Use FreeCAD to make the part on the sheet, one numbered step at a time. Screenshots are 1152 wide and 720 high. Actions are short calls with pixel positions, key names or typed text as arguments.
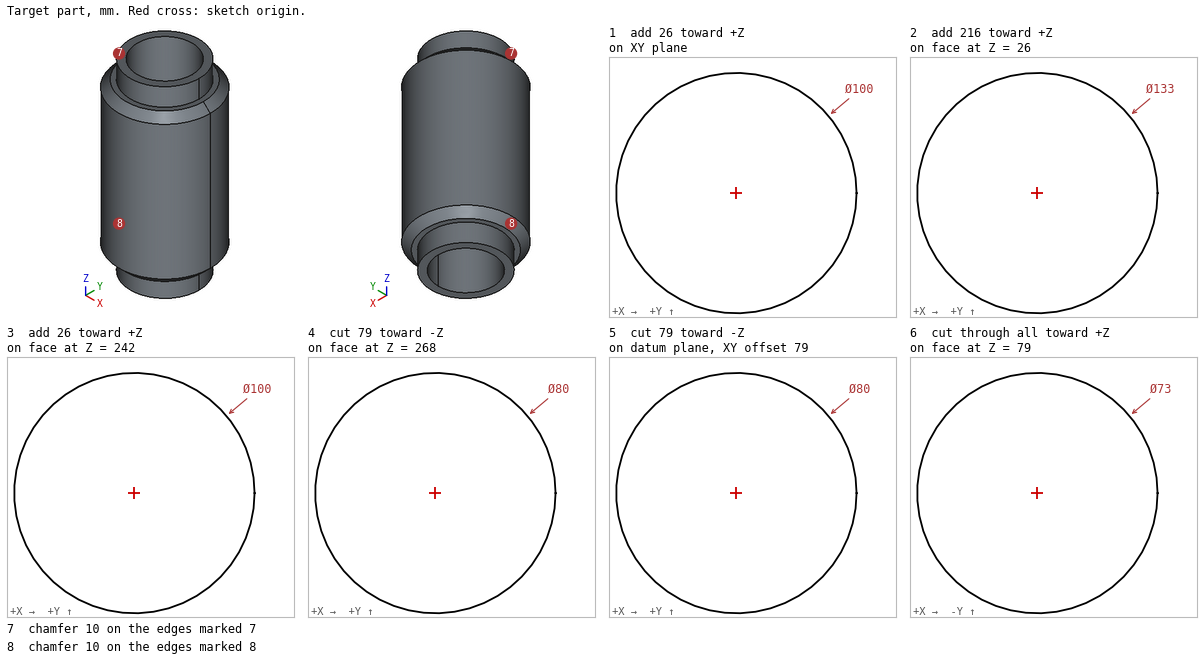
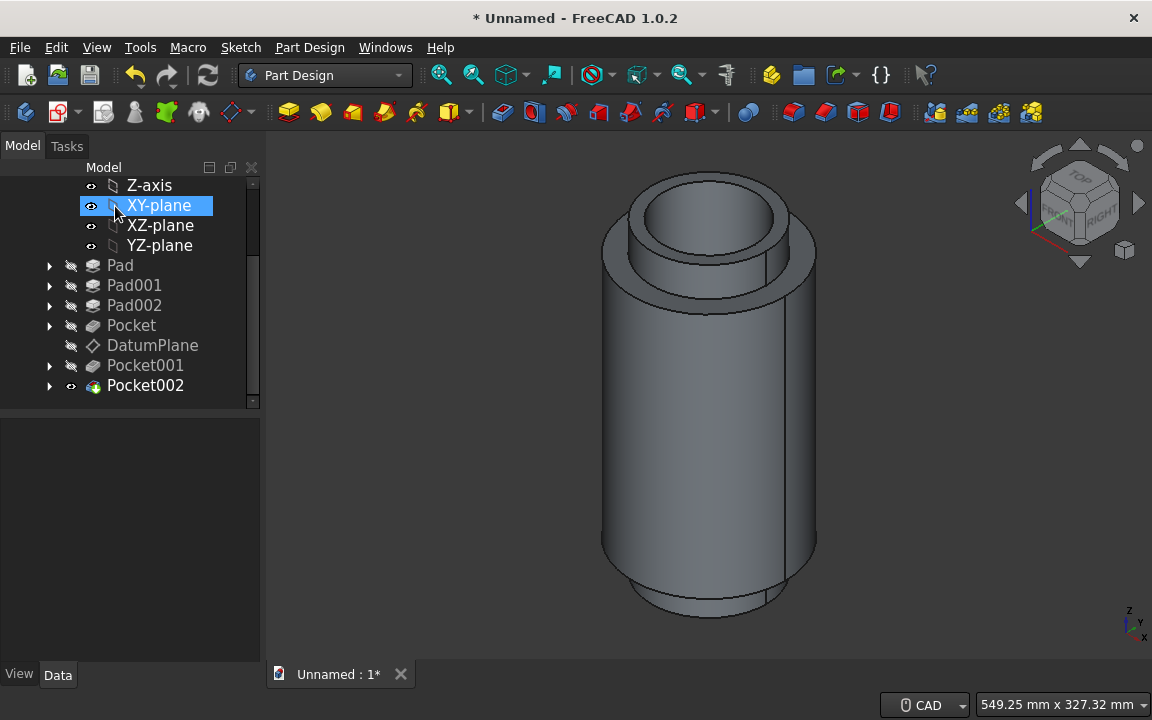
click(613, 280)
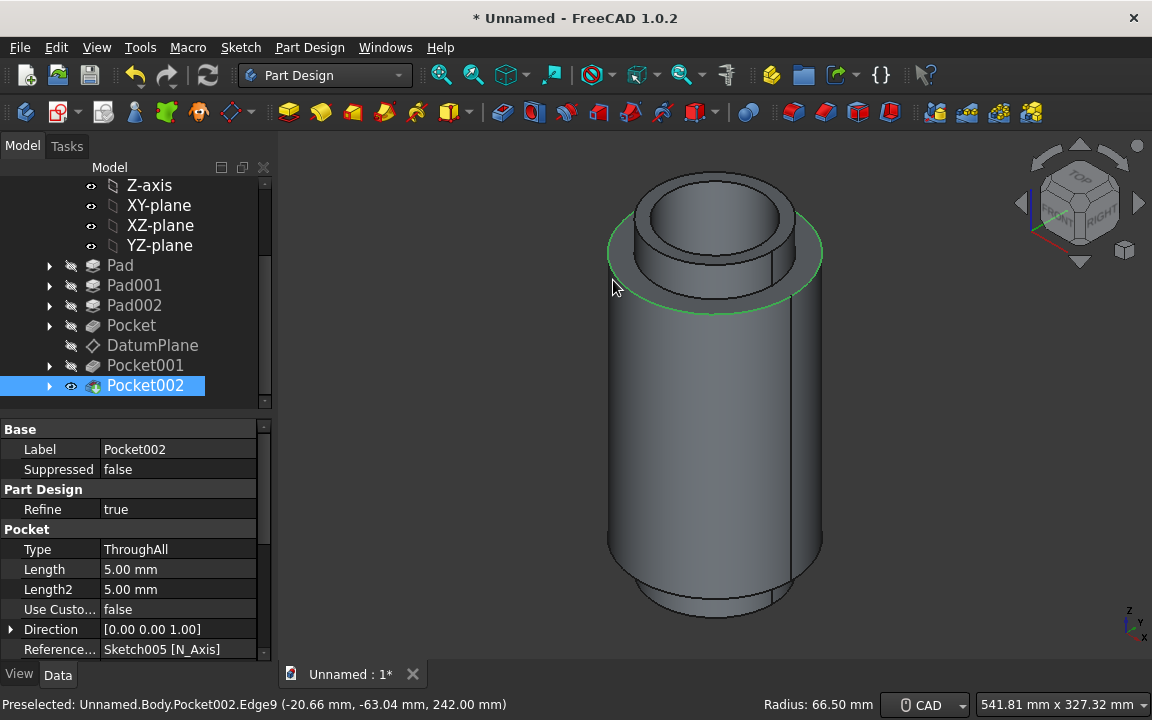
click(826, 112)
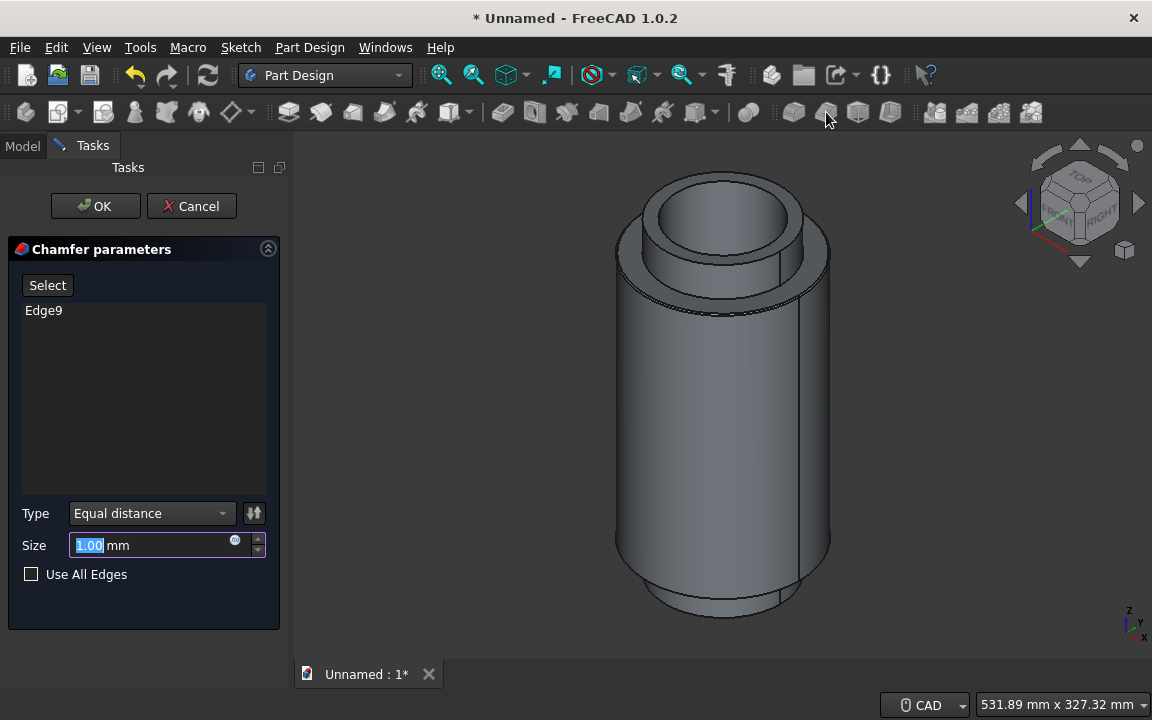
text(10)
key(Tab)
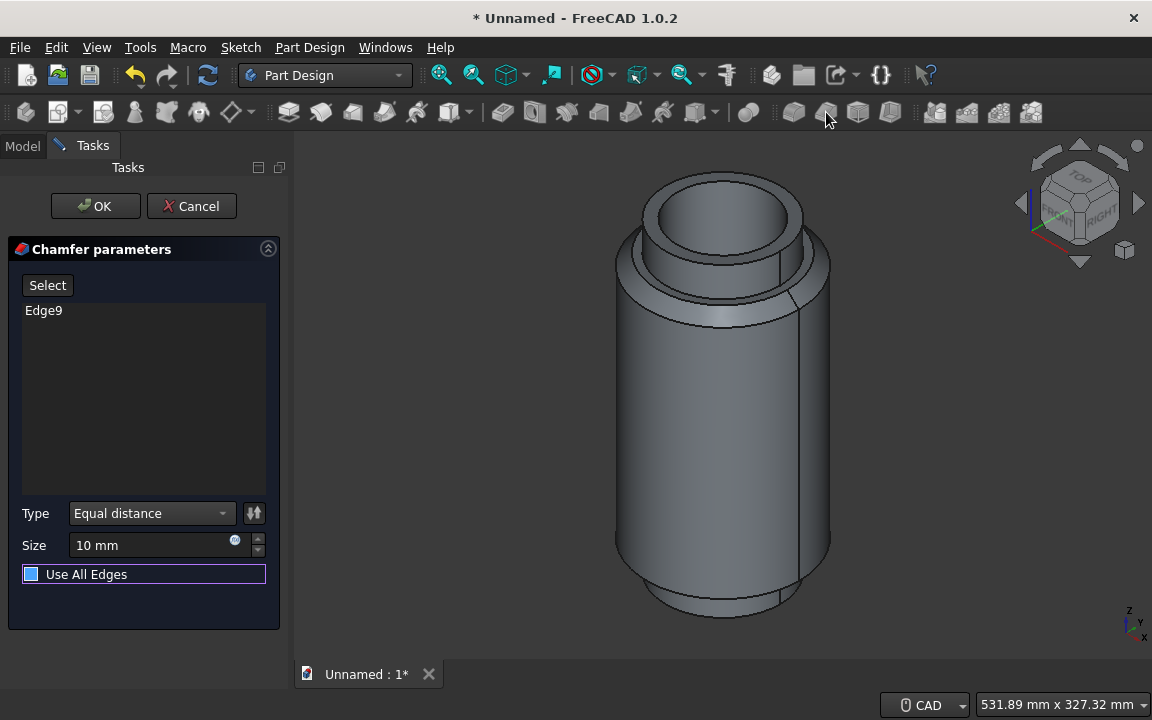
click(96, 206)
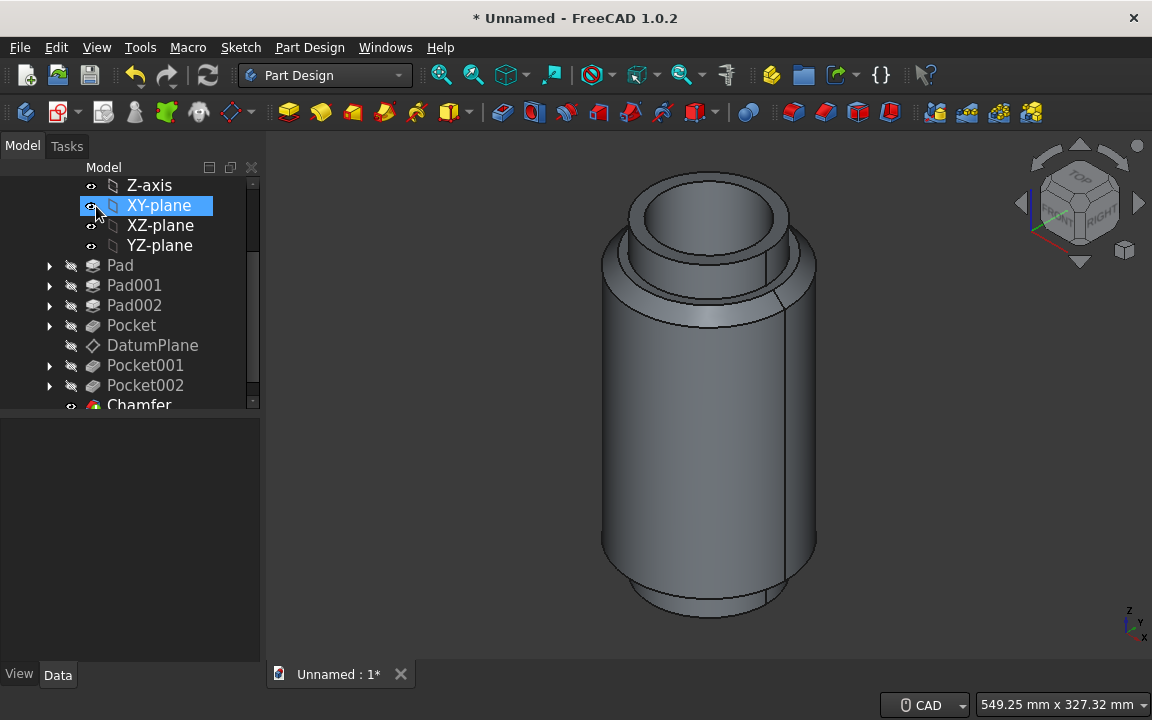
key(v)
key(f)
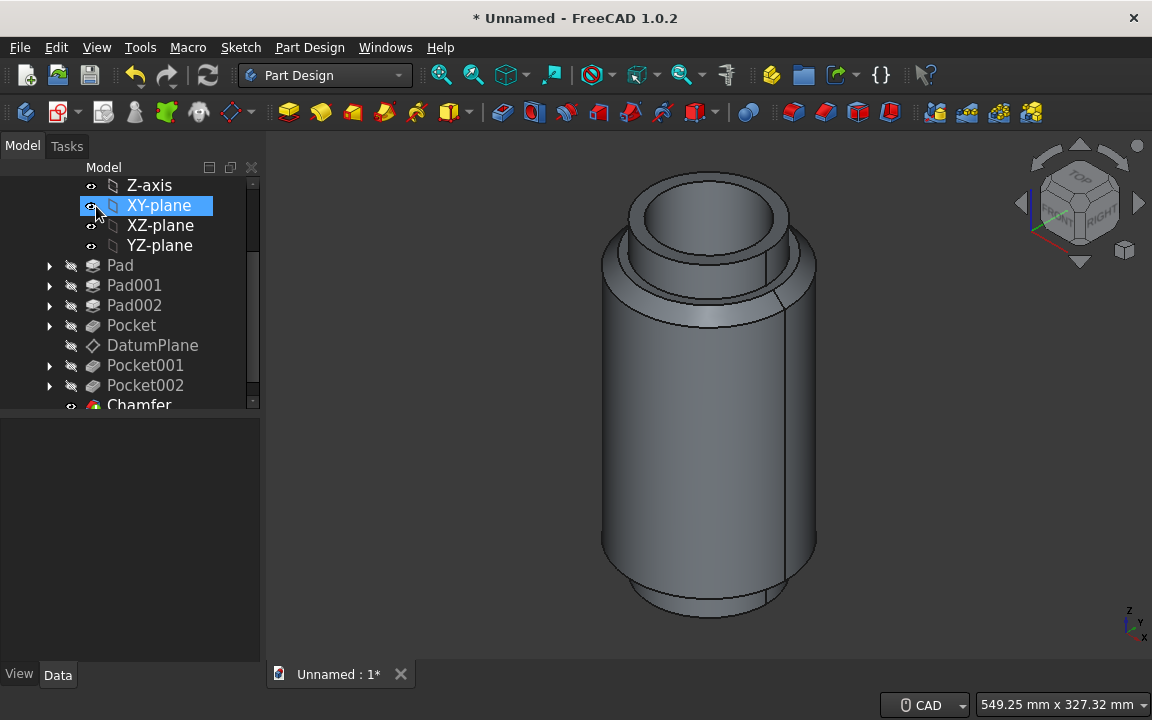
key(2)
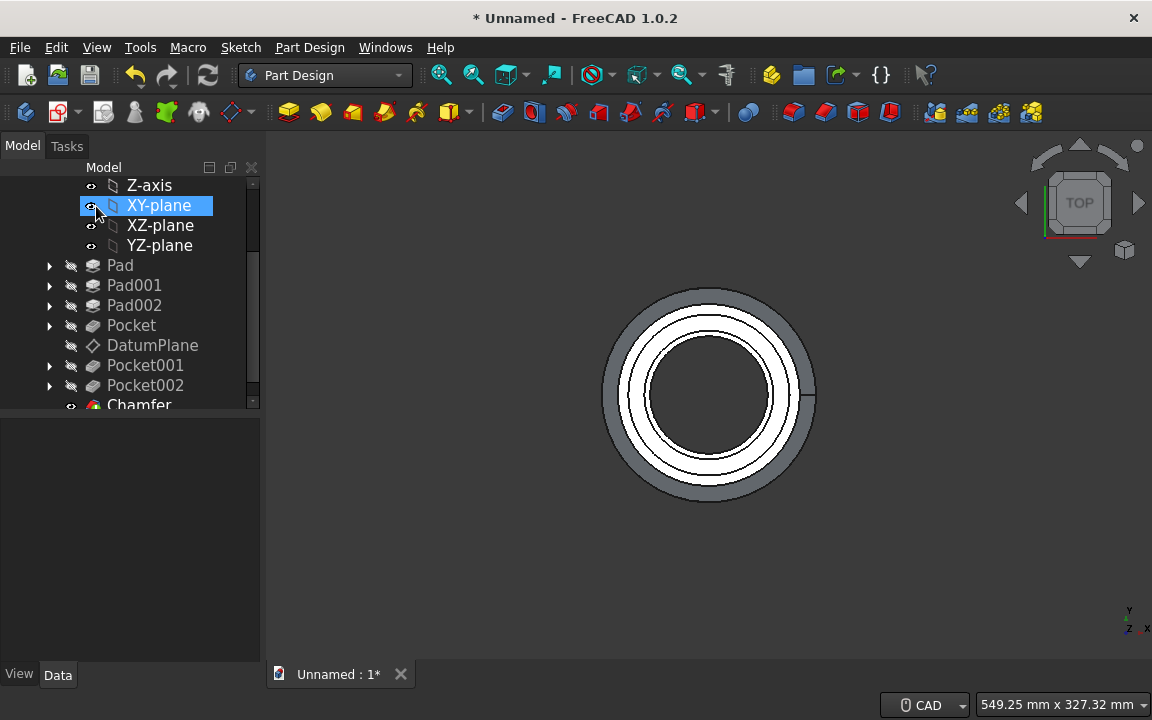
key(v)
key(f)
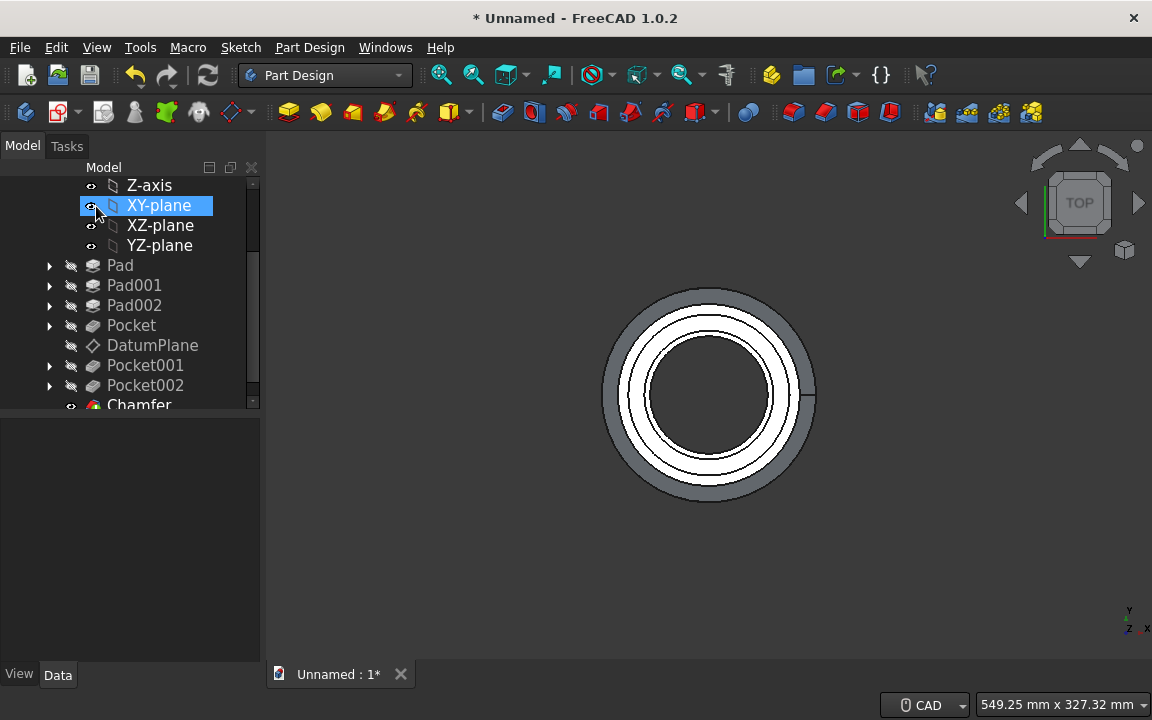
key(0)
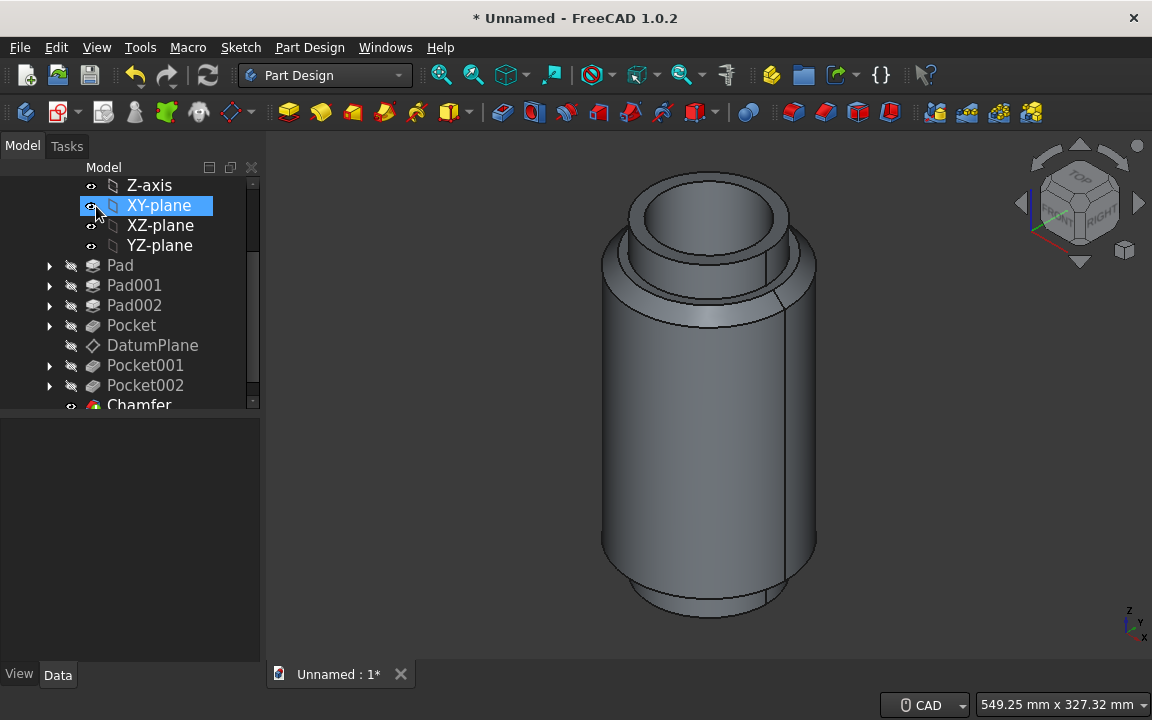
key(v)
key(f)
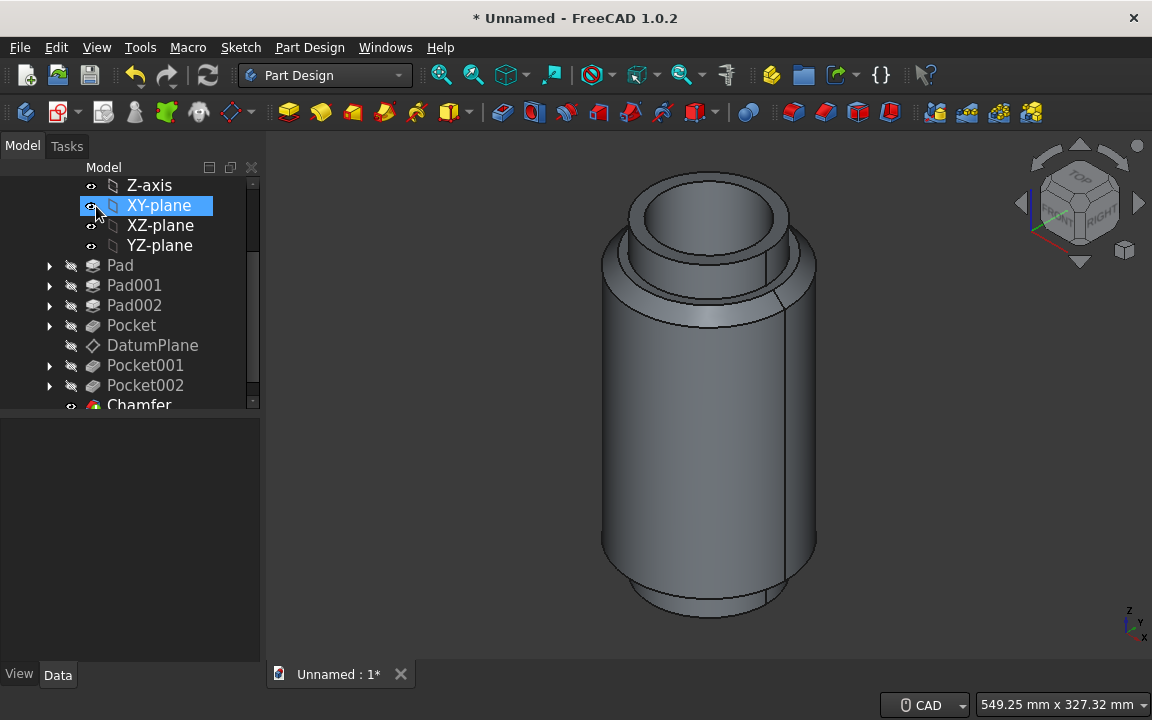
key(1)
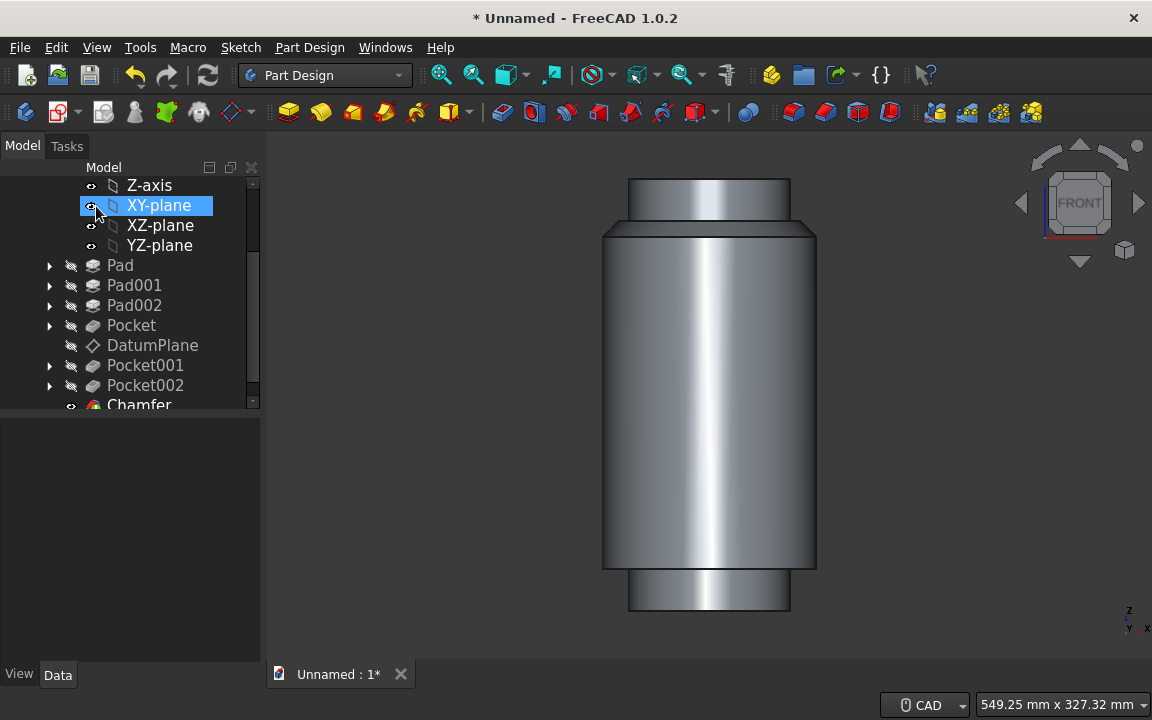
key(3)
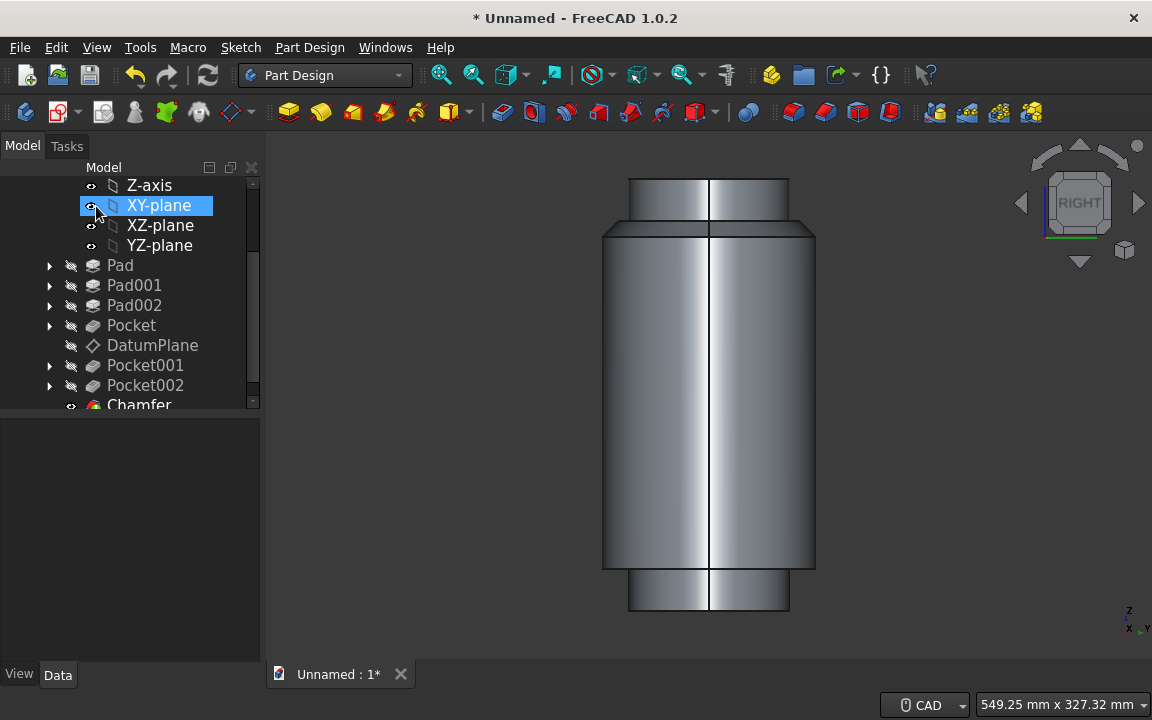
key(5)